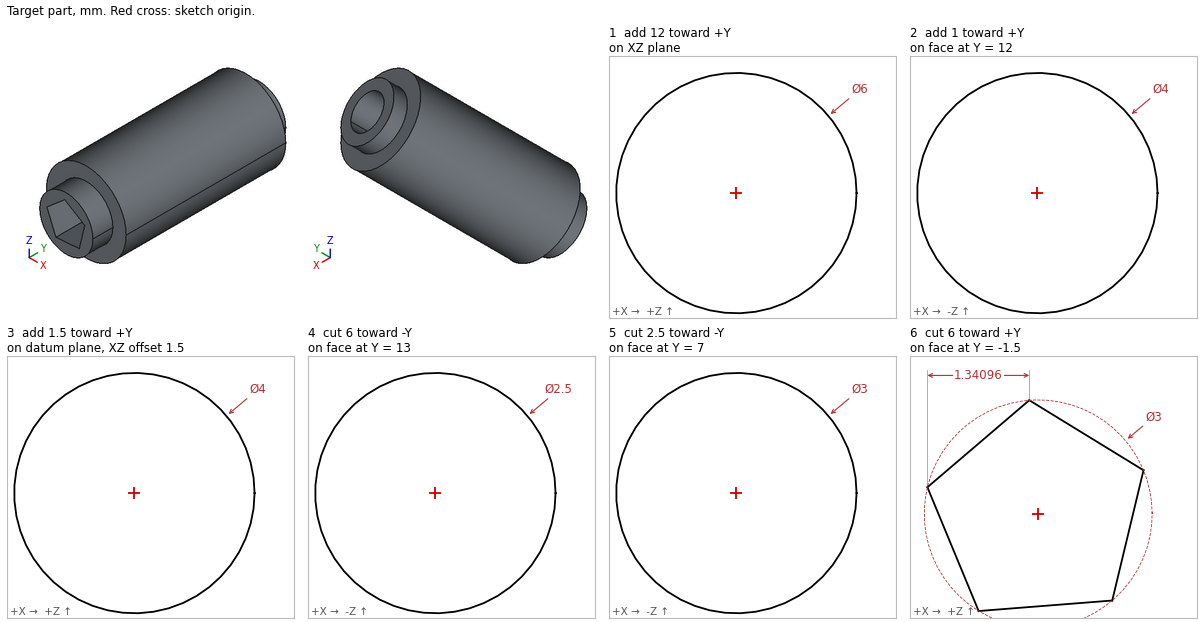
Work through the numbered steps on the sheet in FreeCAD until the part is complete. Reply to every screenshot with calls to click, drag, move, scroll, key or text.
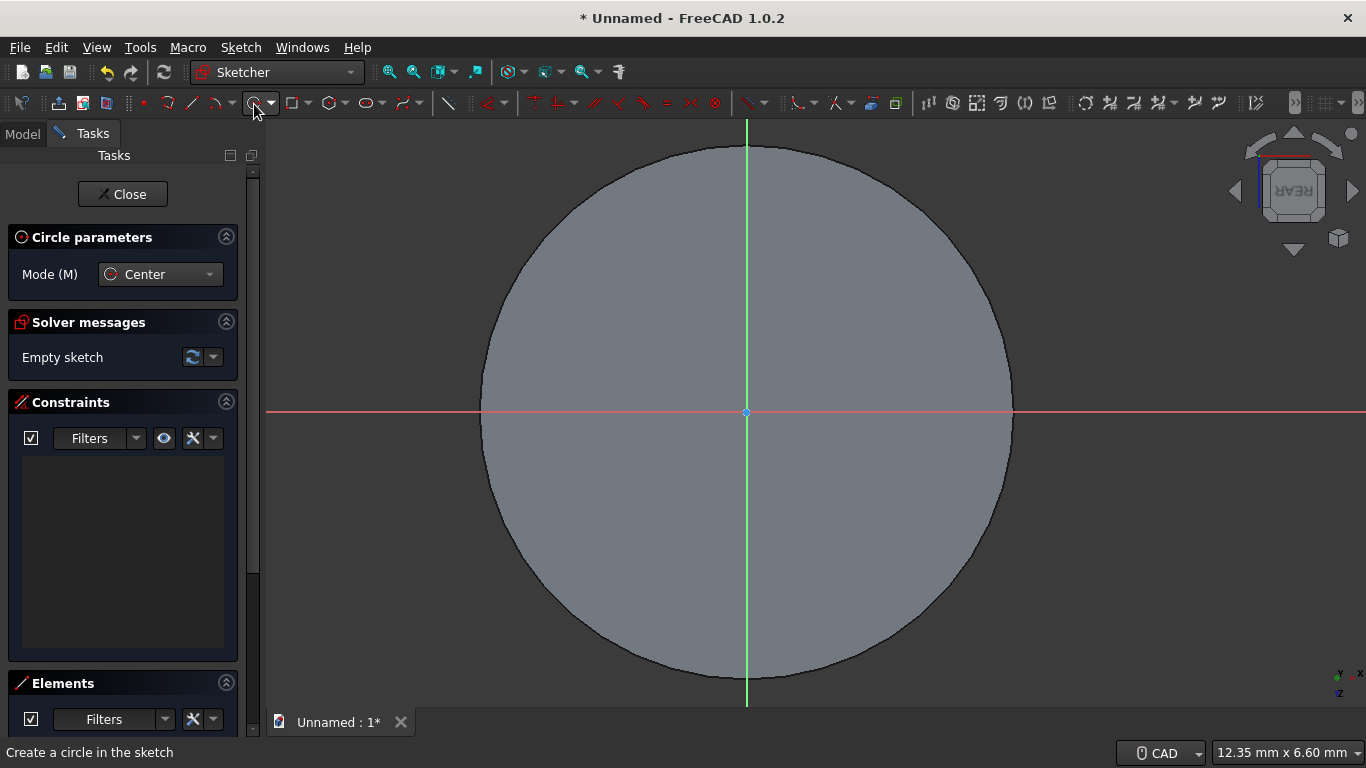
click(747, 412)
move(873, 286)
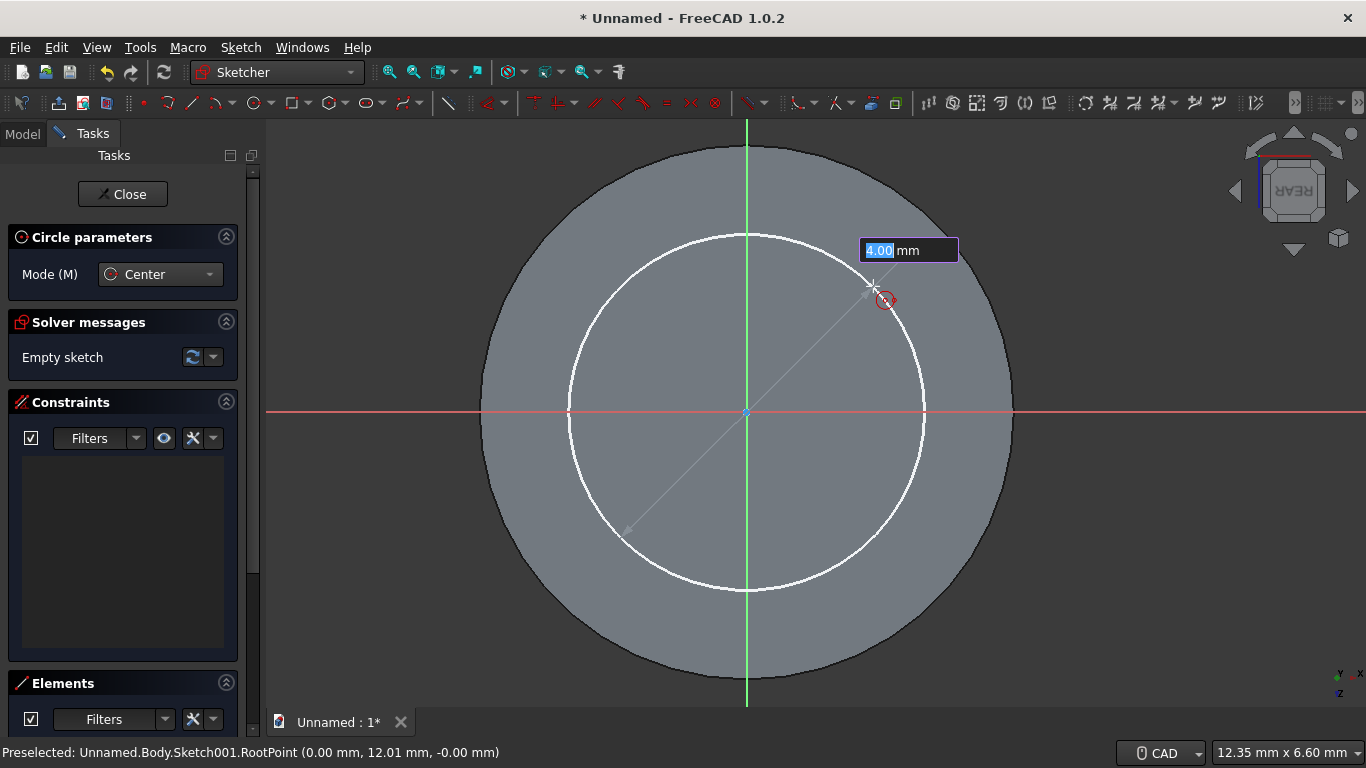
text(4)
key(Return)
key(Escape)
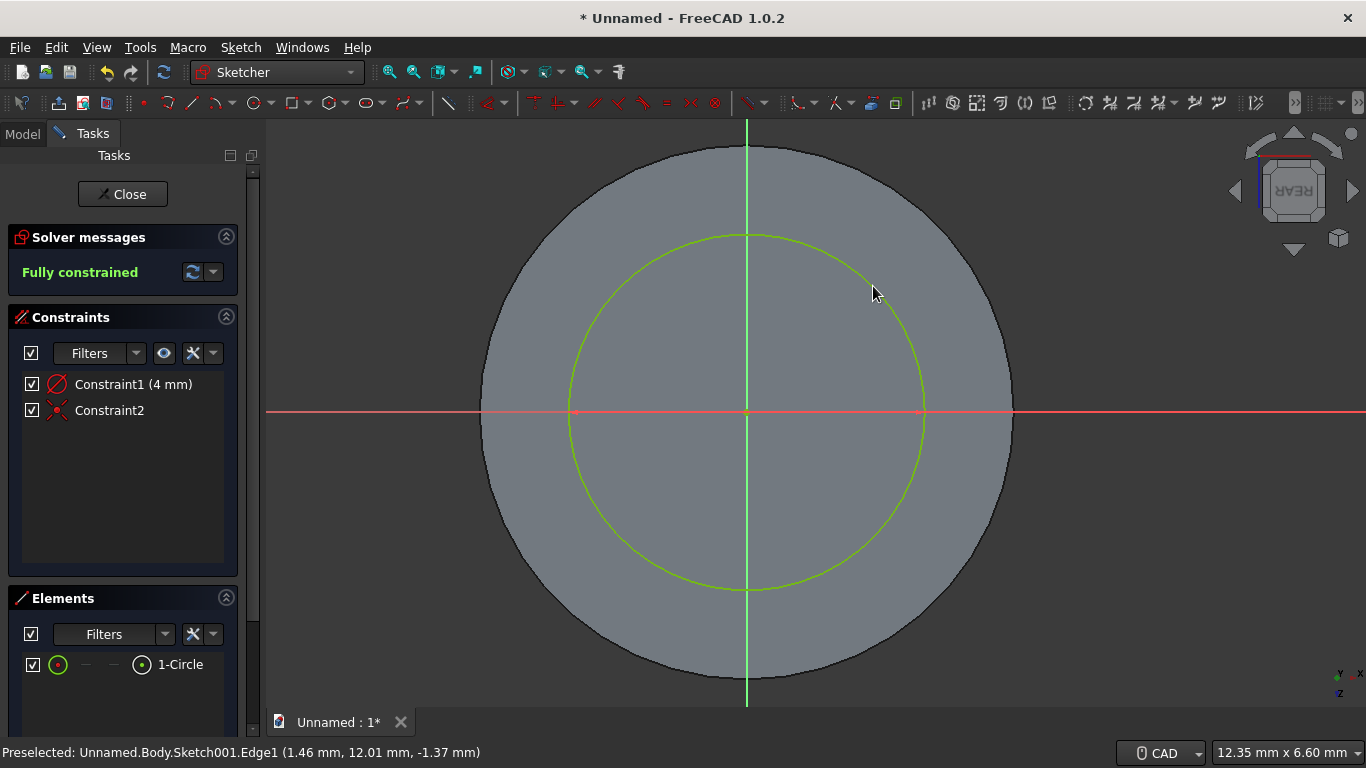
click(123, 194)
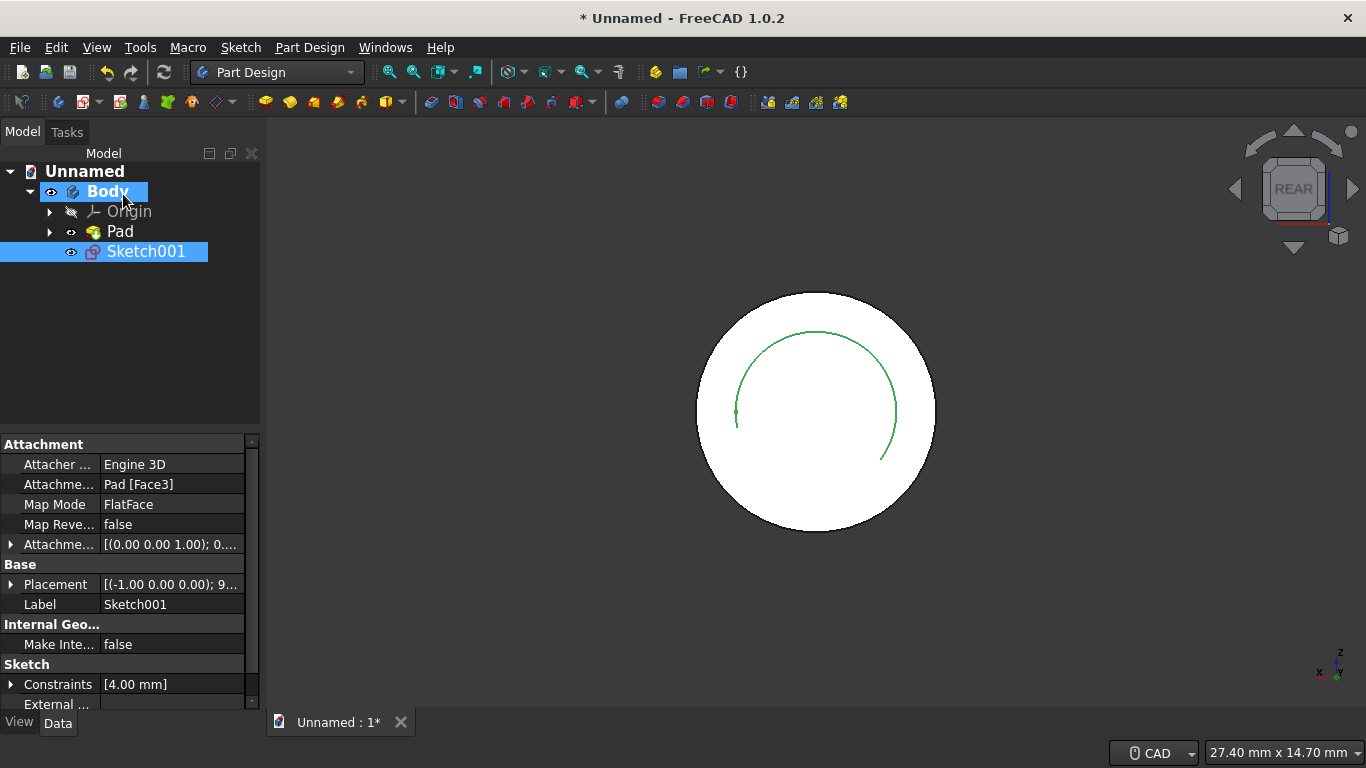
click(266, 102)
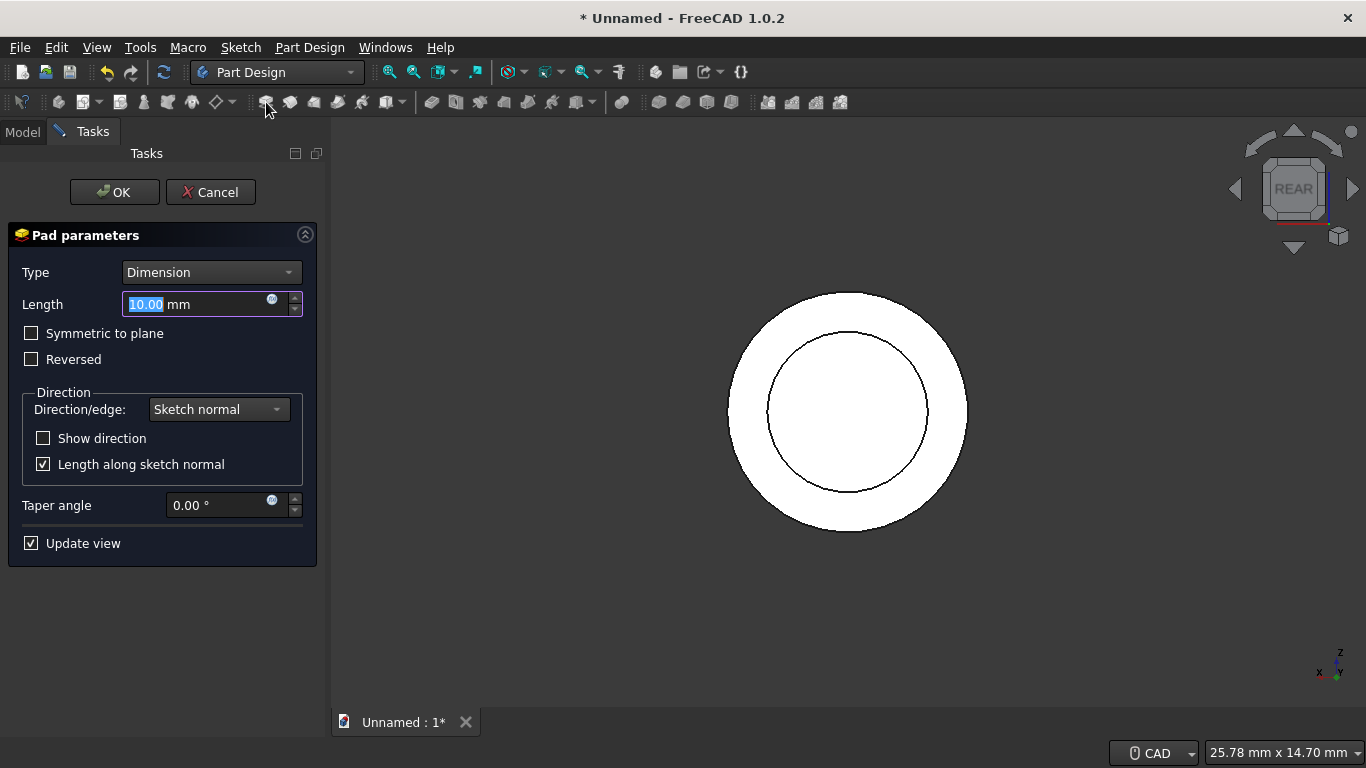
text(1)
key(Tab)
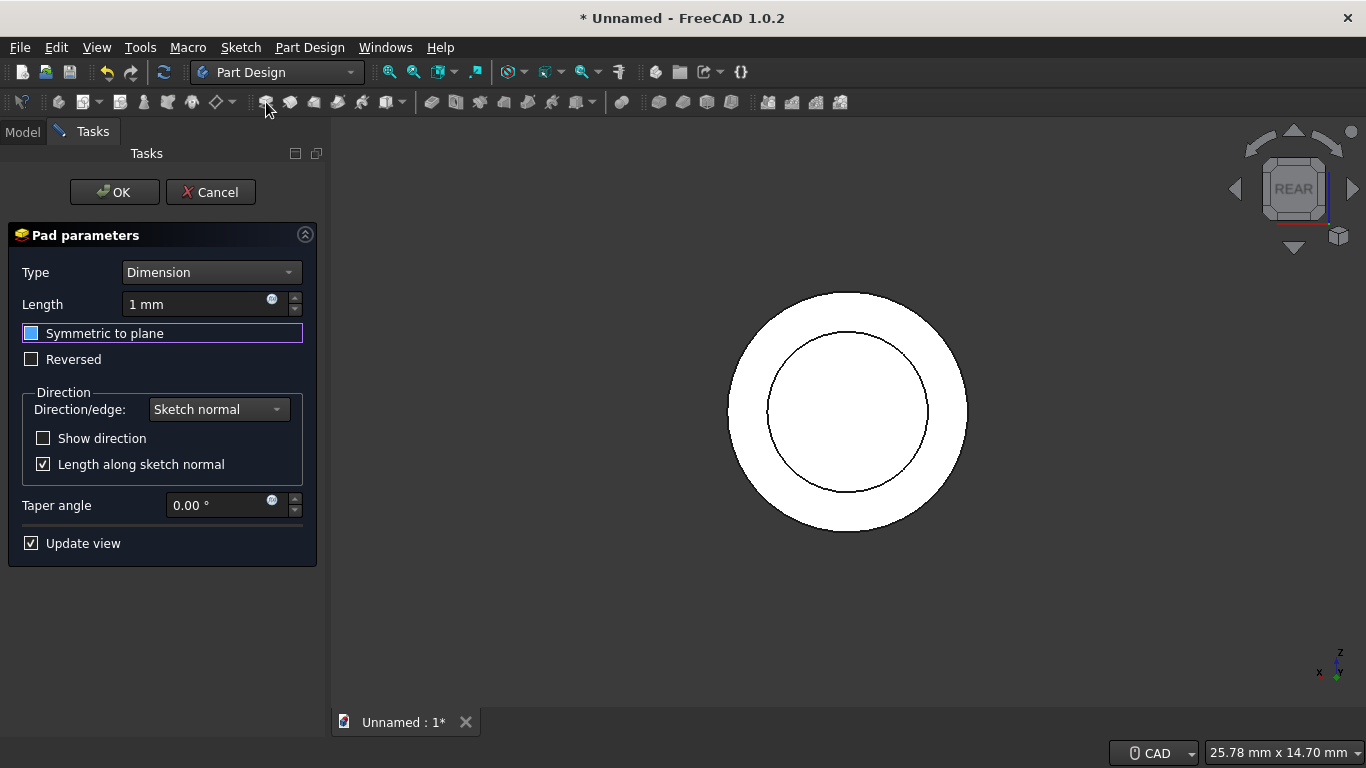
click(115, 192)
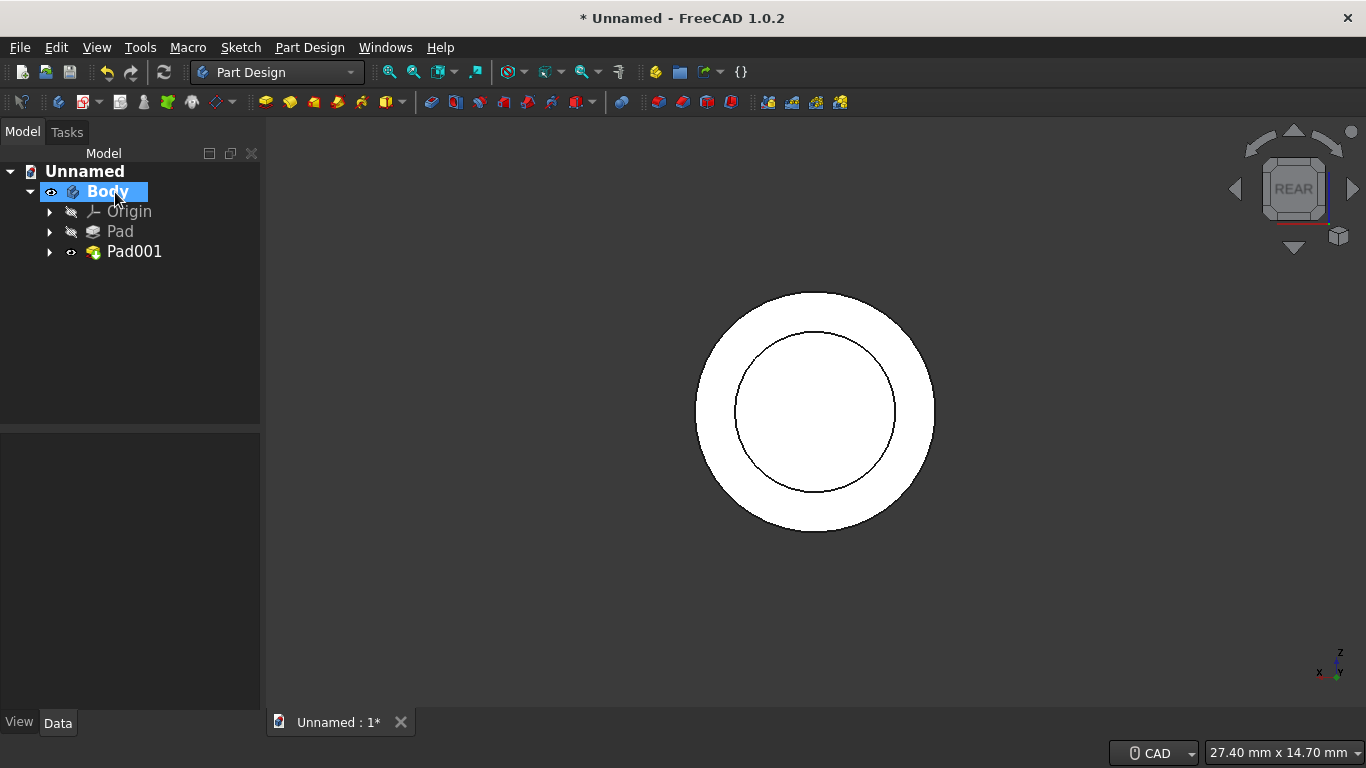
click(390, 72)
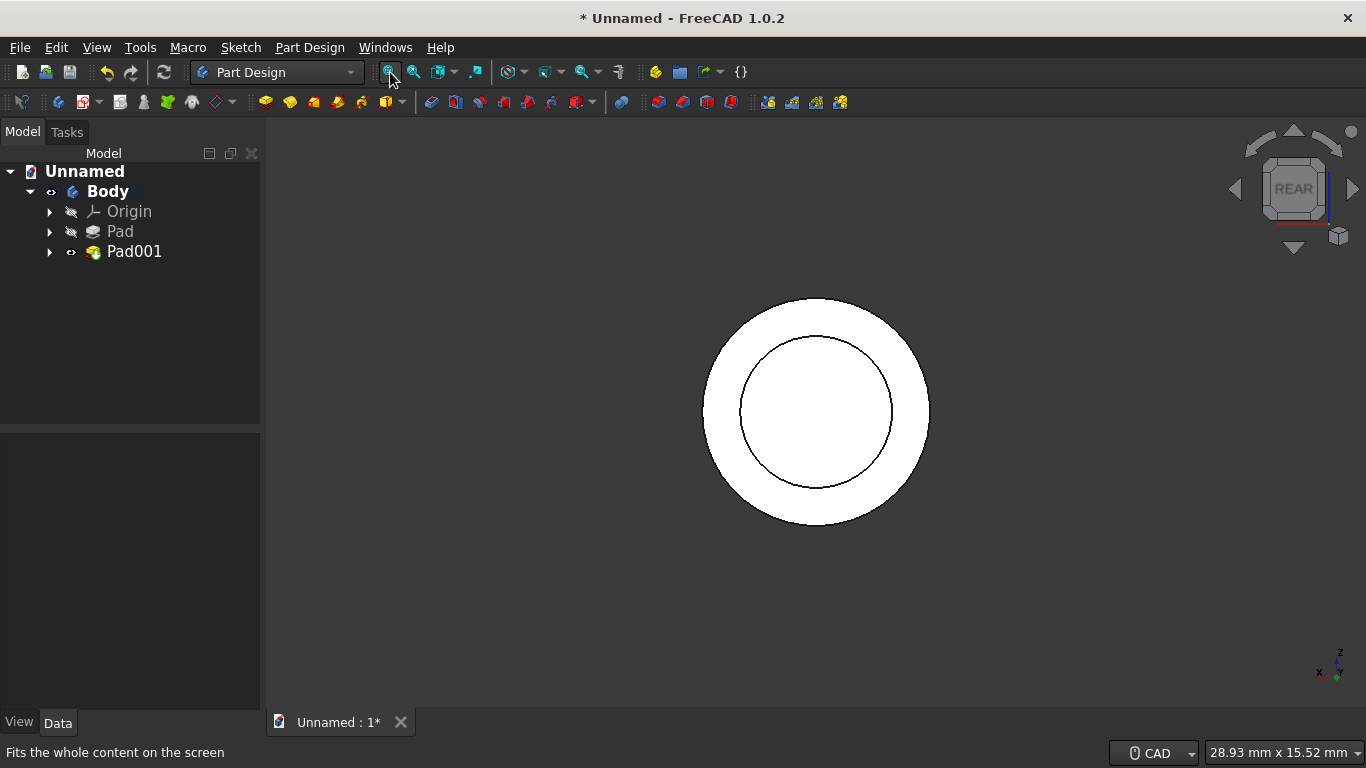
click(50, 212)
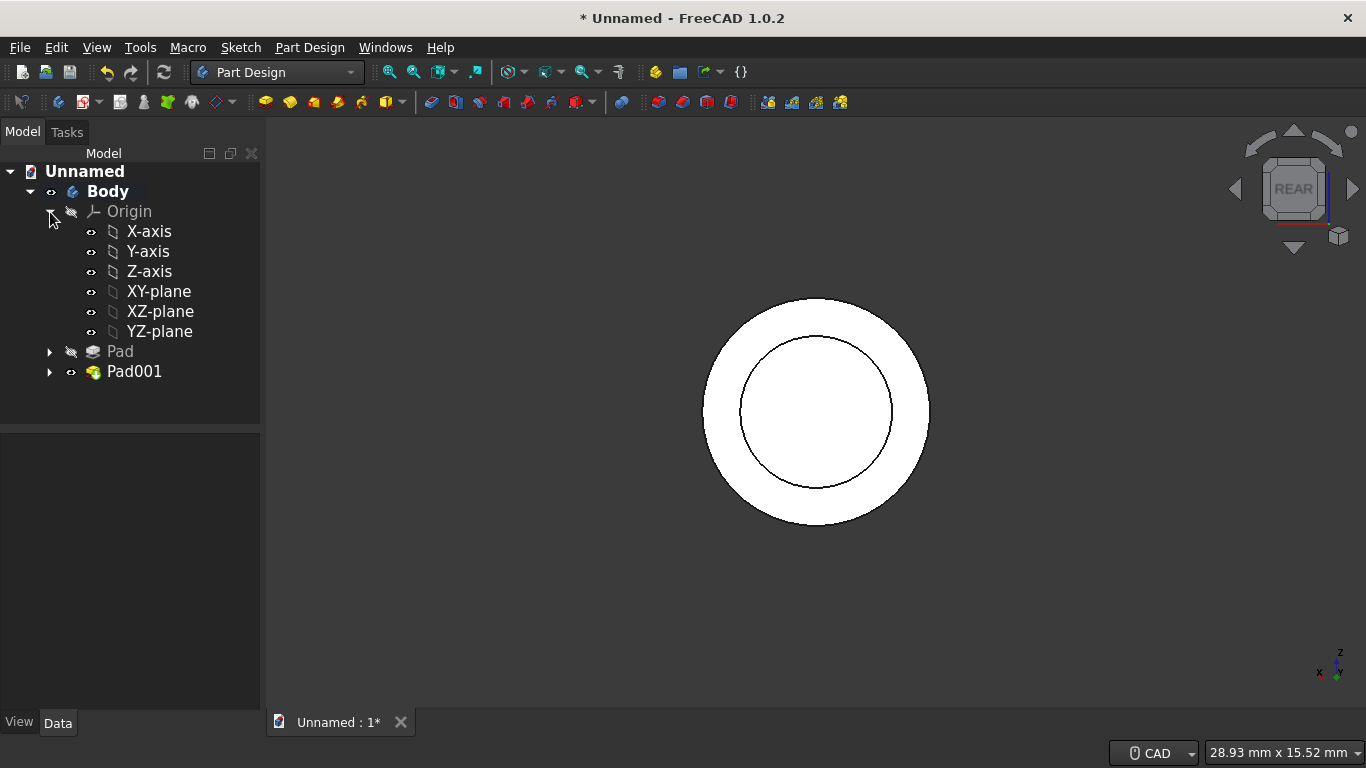
click(136, 312)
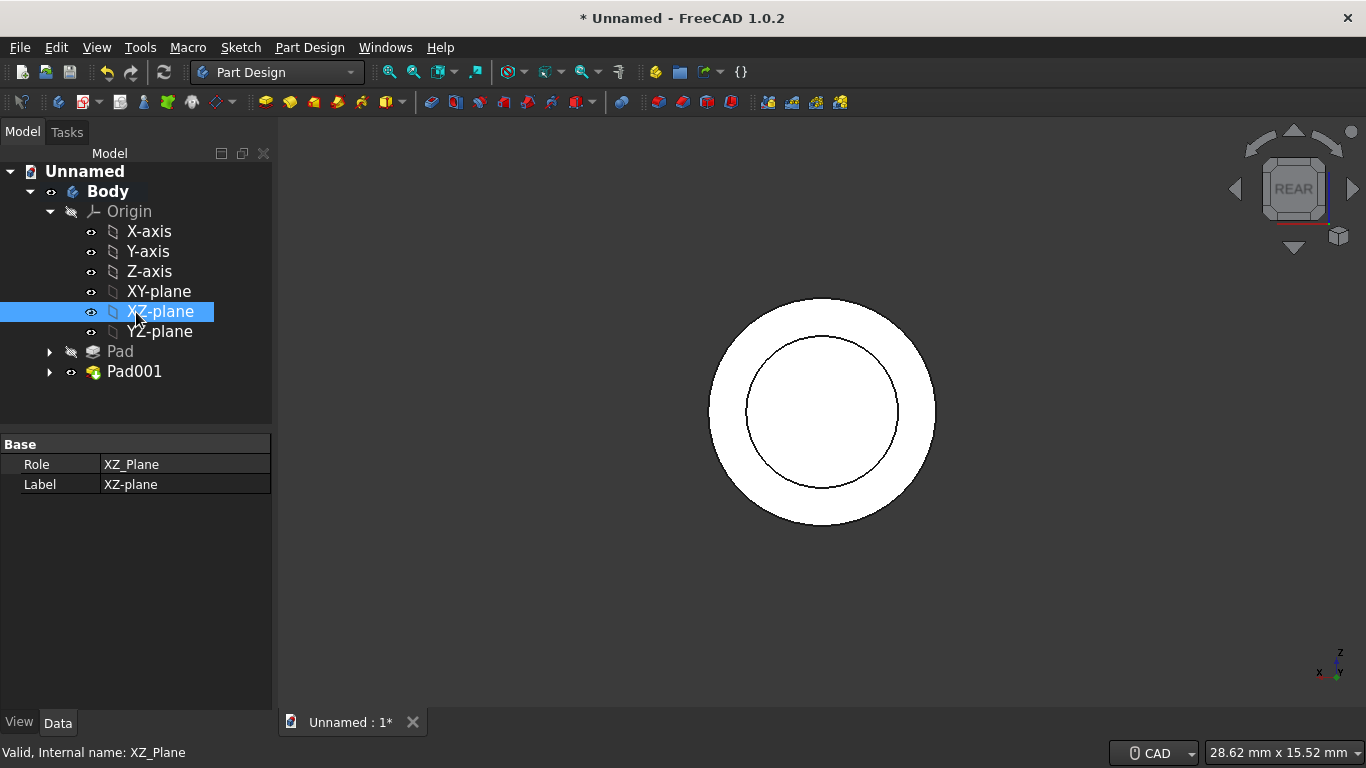
click(216, 102)